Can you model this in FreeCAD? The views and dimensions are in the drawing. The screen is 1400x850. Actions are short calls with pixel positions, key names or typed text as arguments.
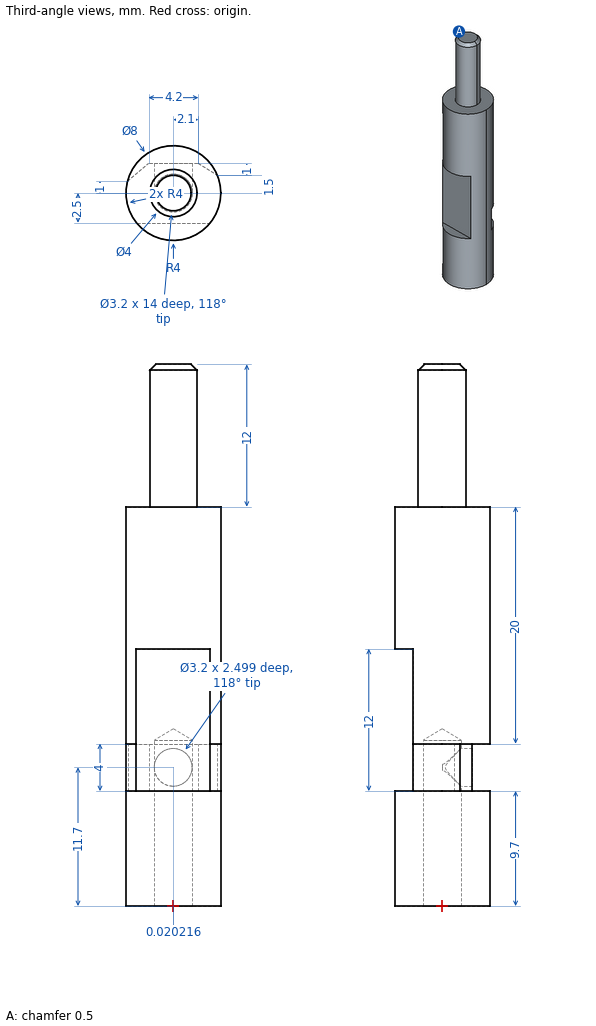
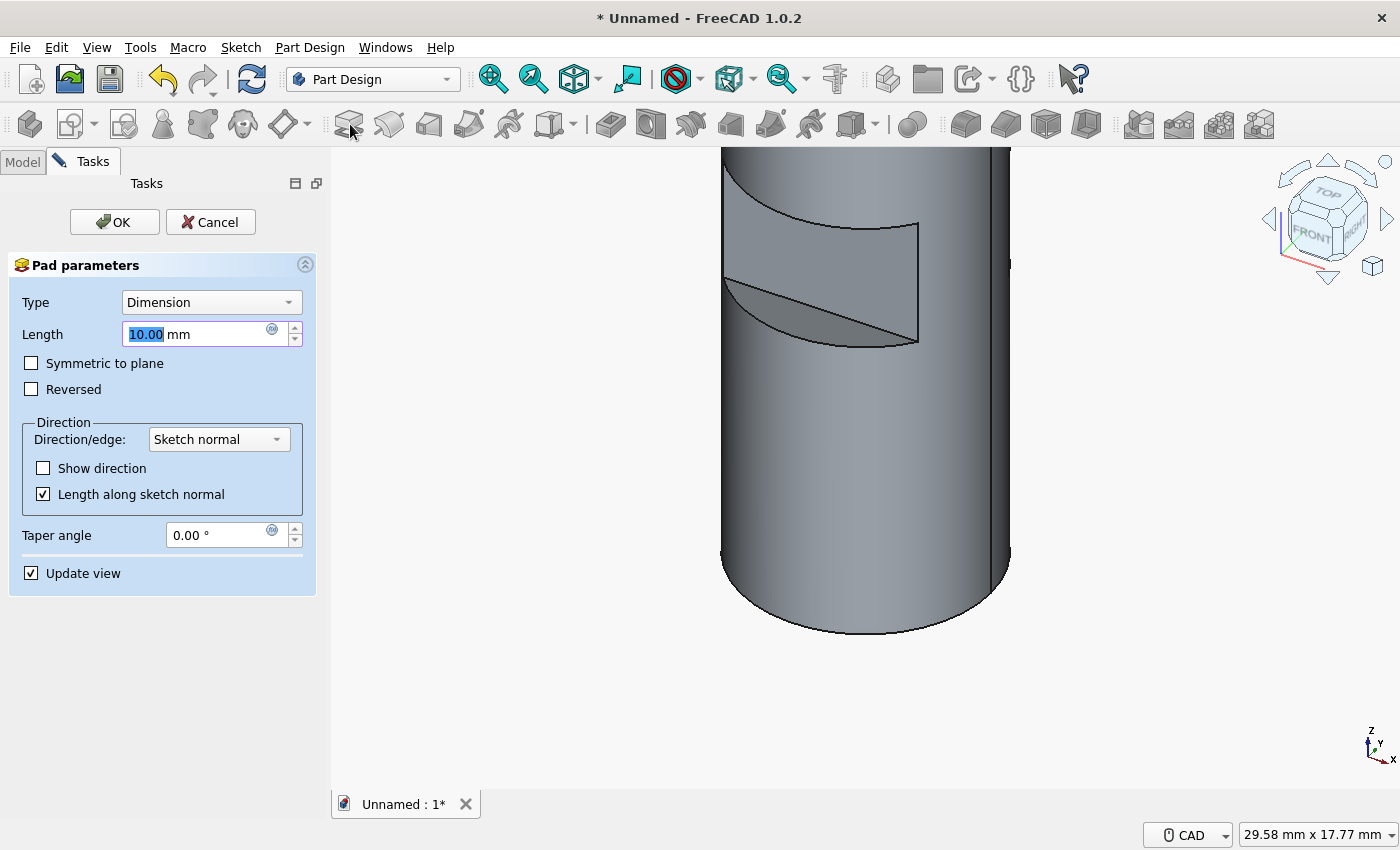
text(20)
key(Tab)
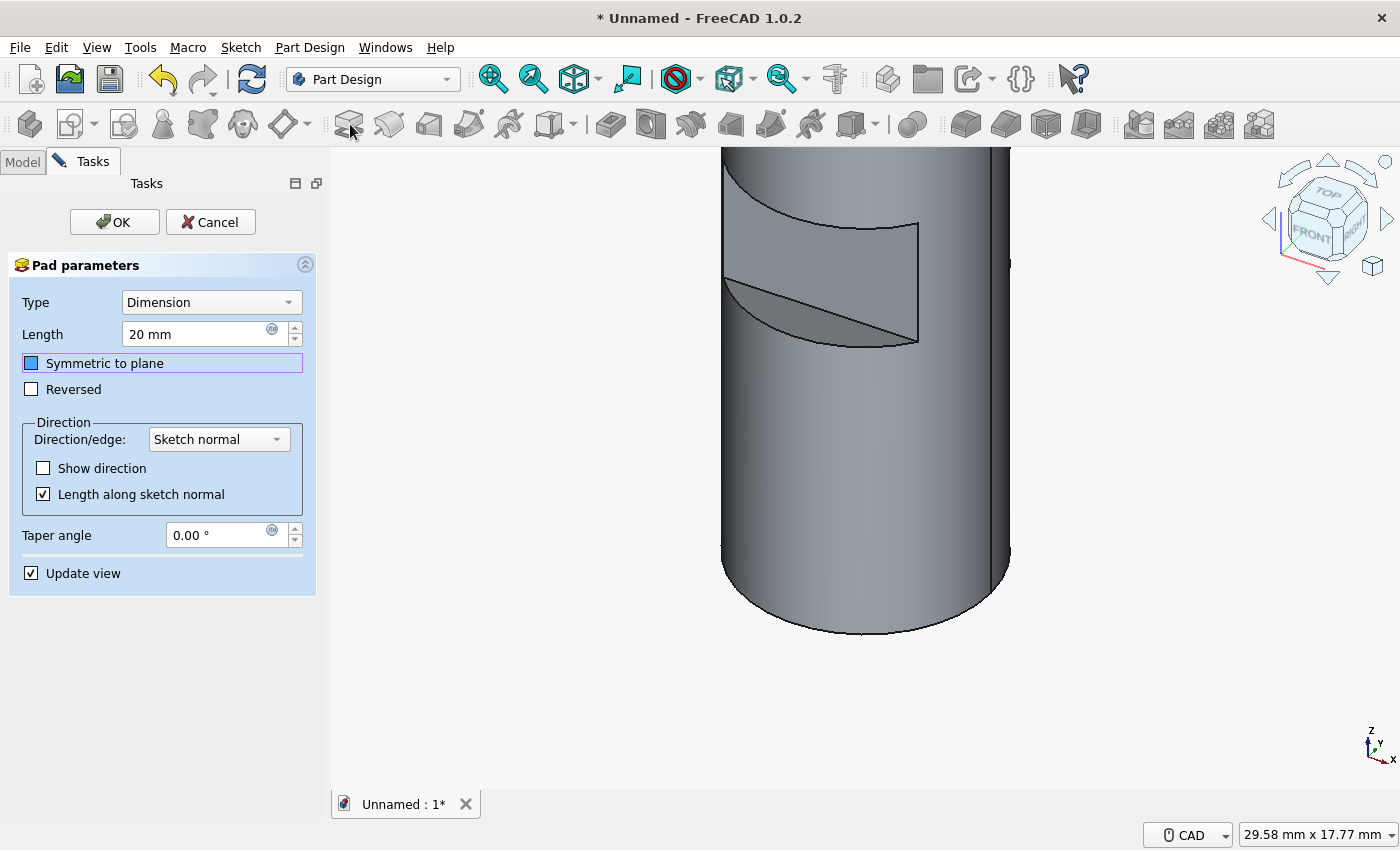
click(115, 222)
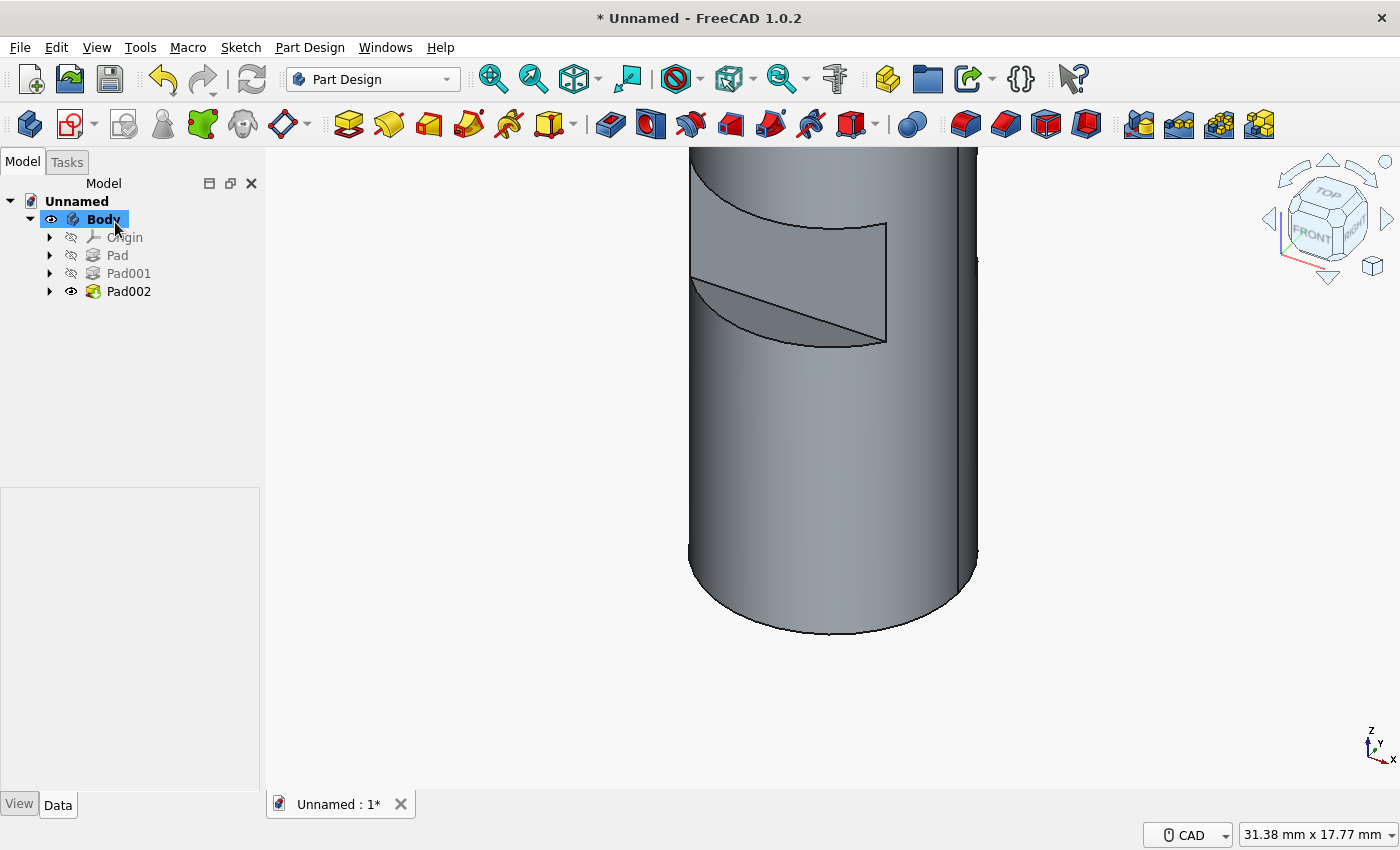
click(494, 80)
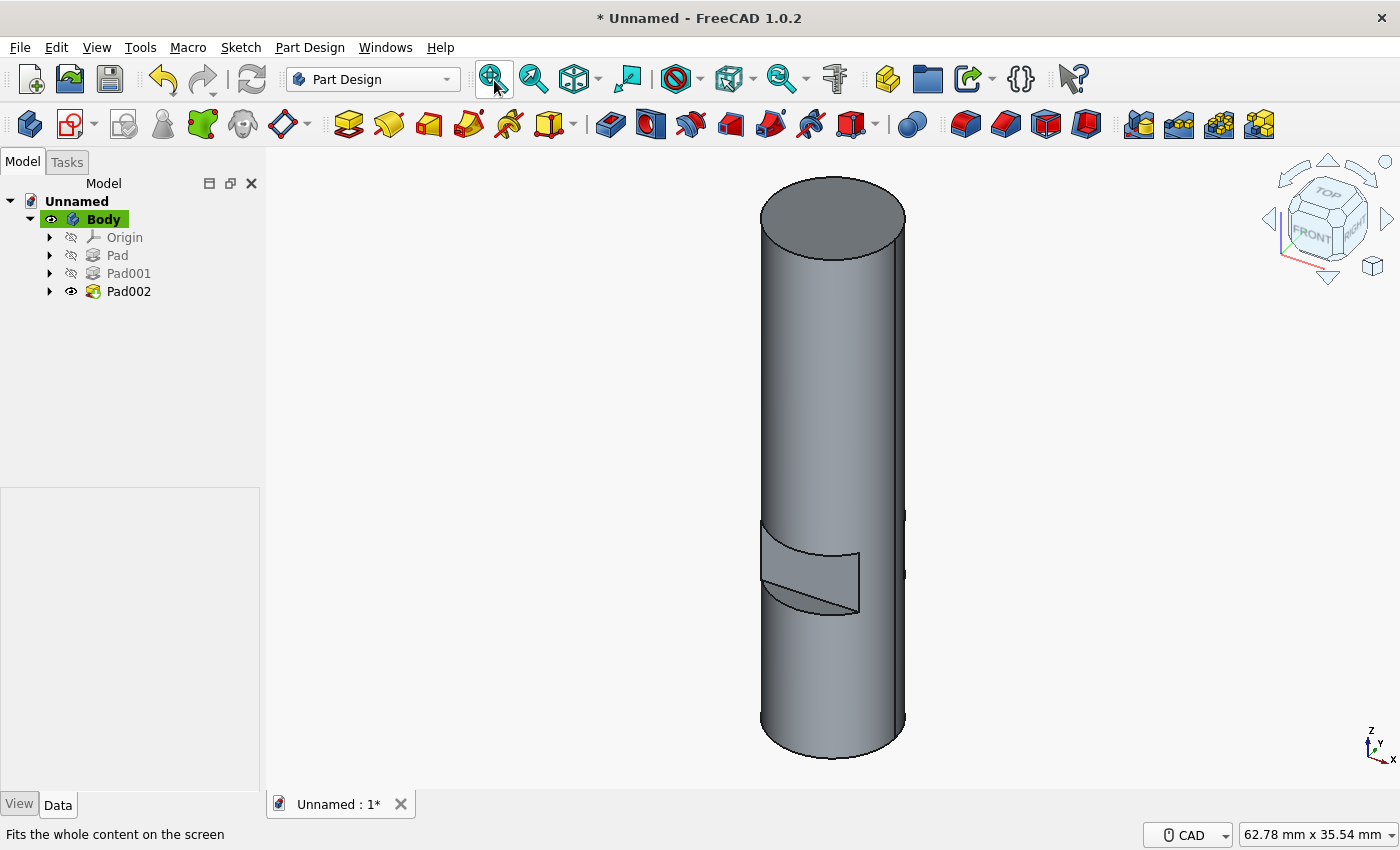
click(833, 218)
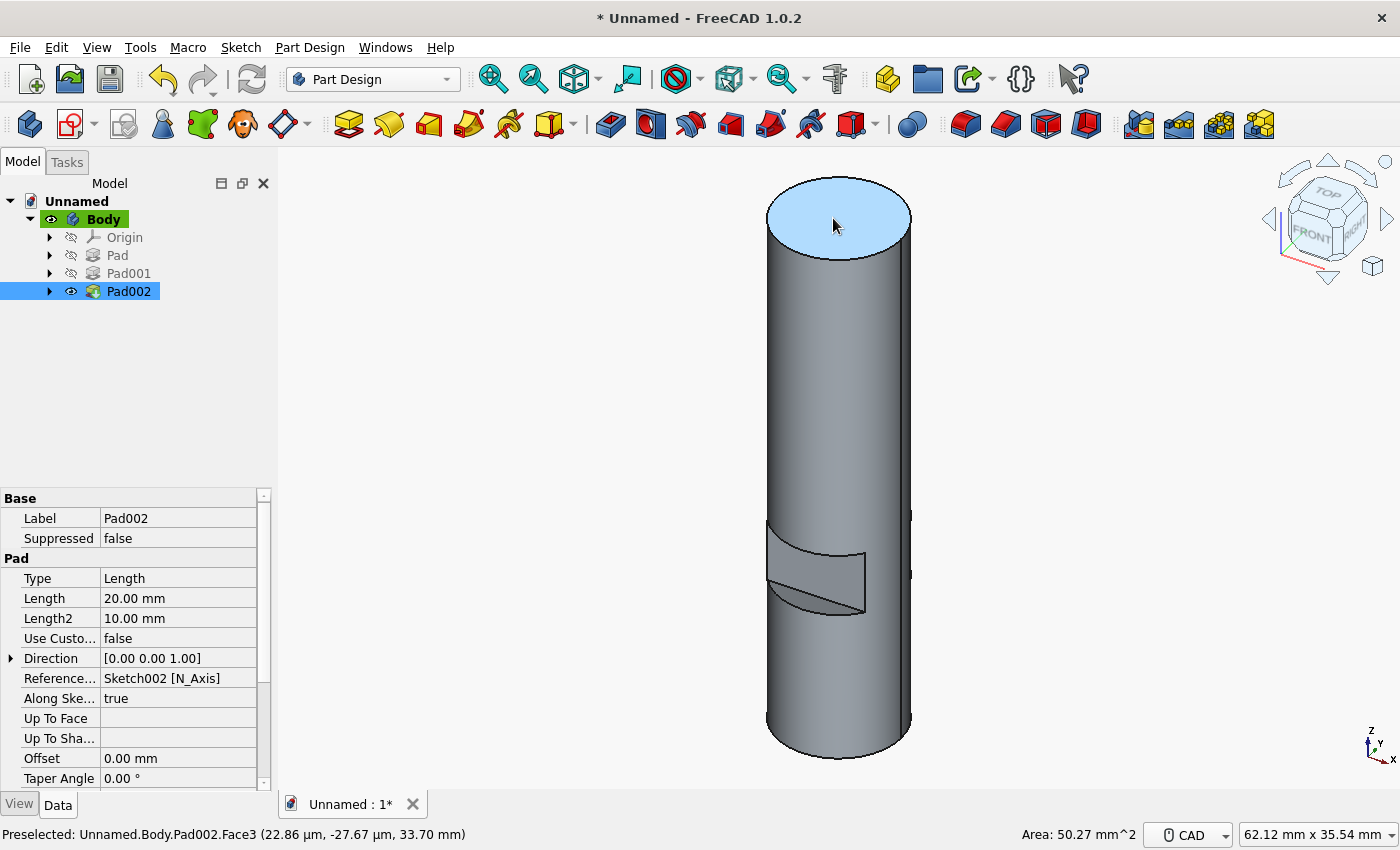
click(70, 124)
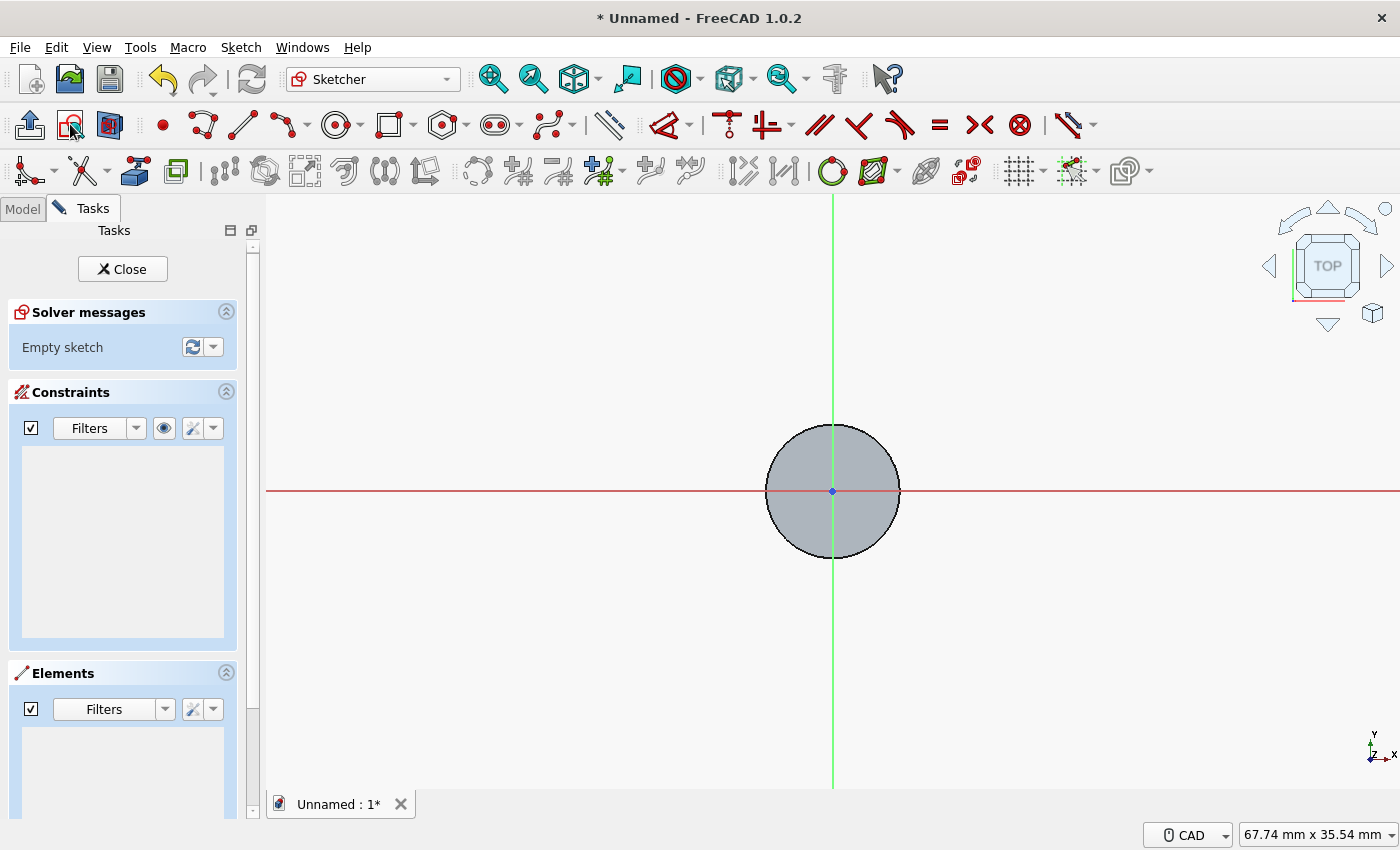
scroll(846, 491, up, 9)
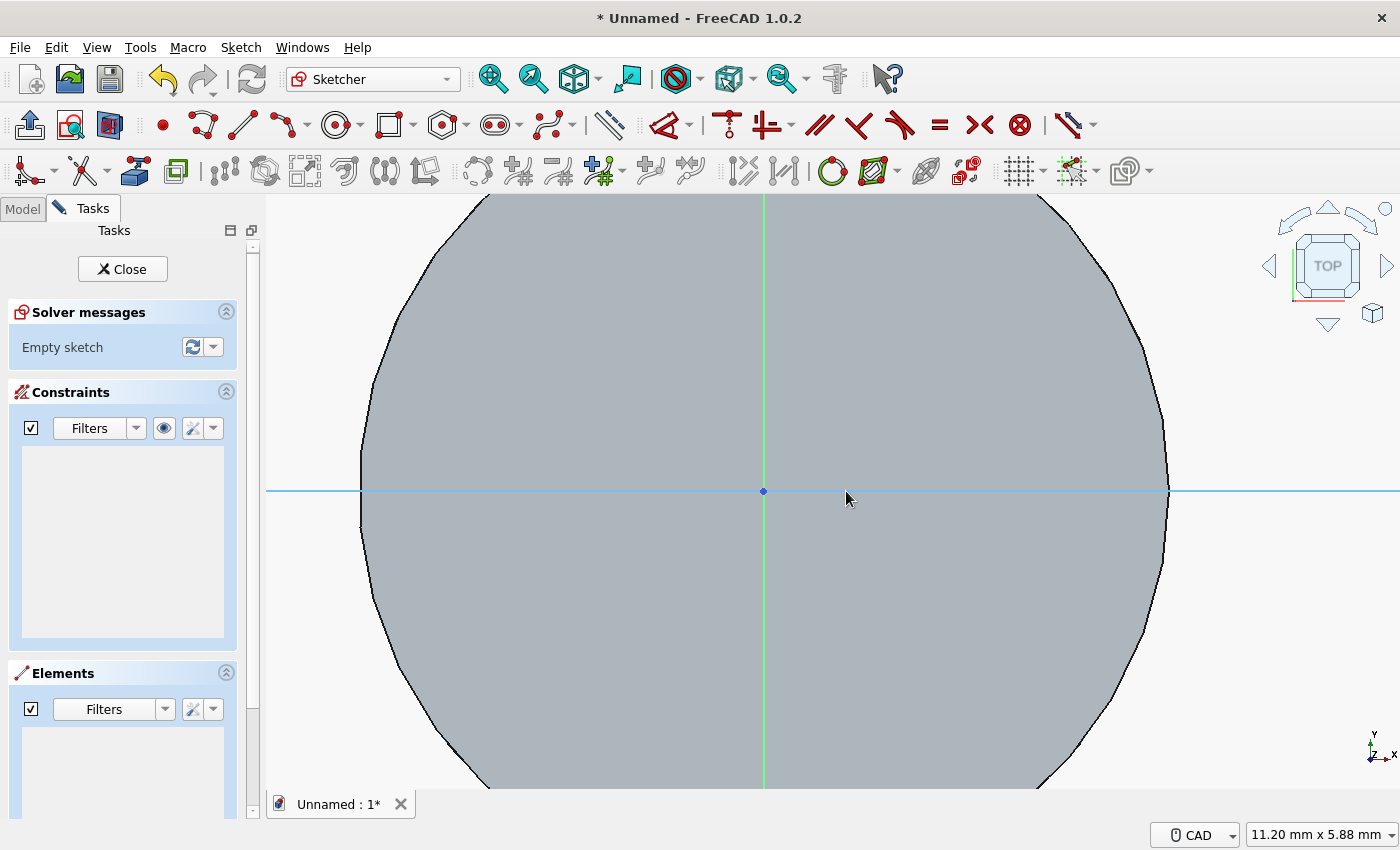
click(336, 126)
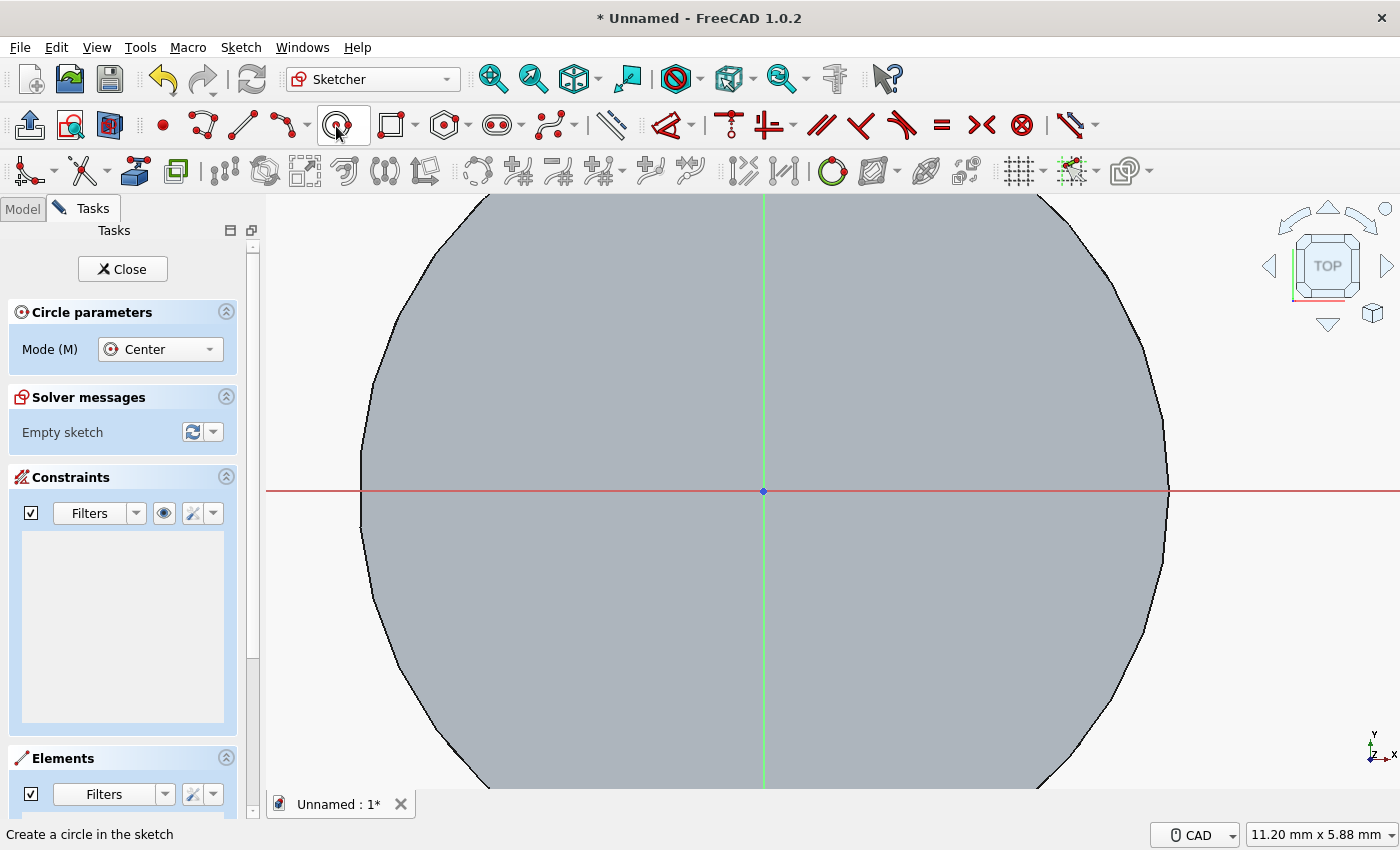
click(764, 491)
click(907, 348)
key(Escape)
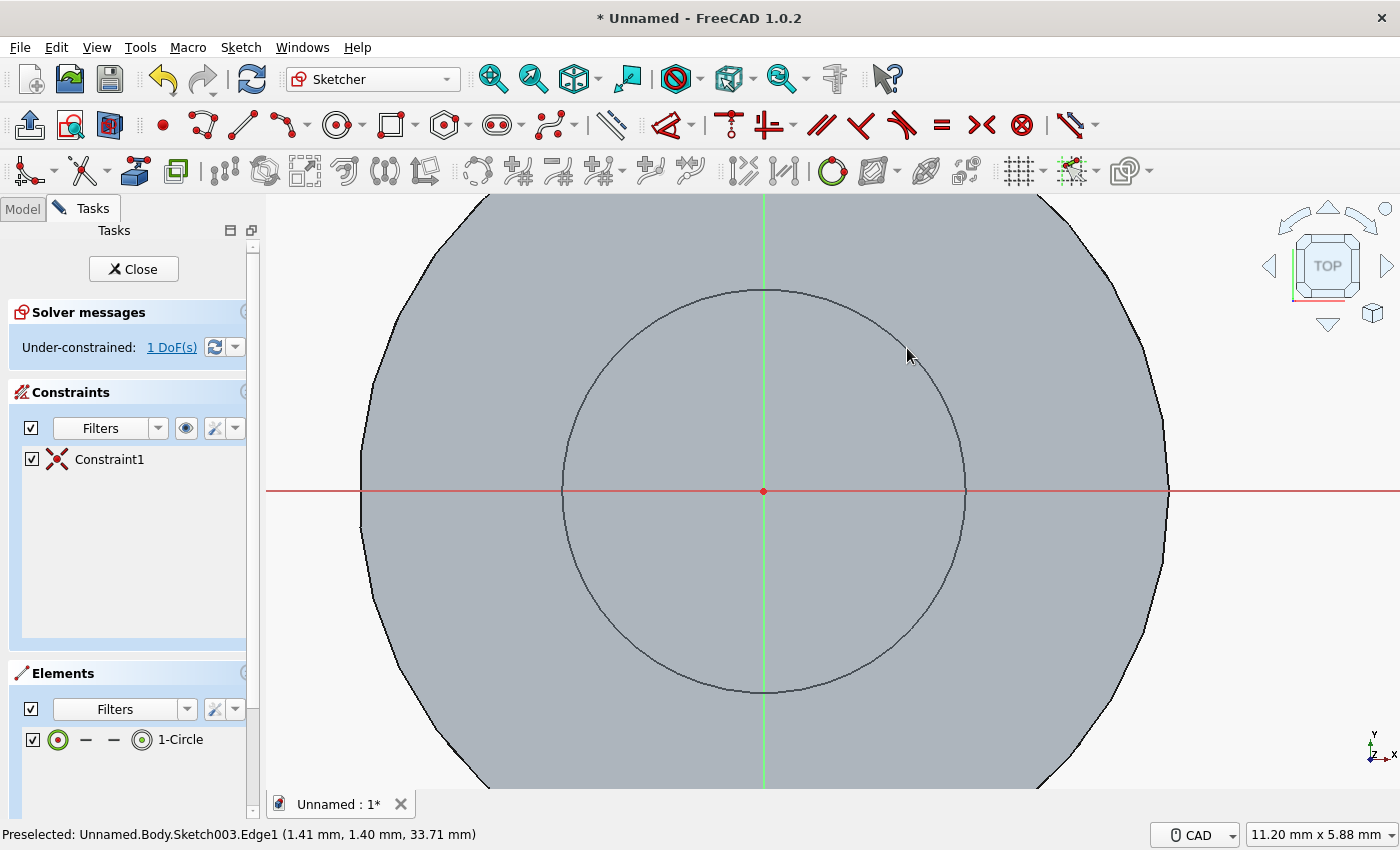
click(666, 126)